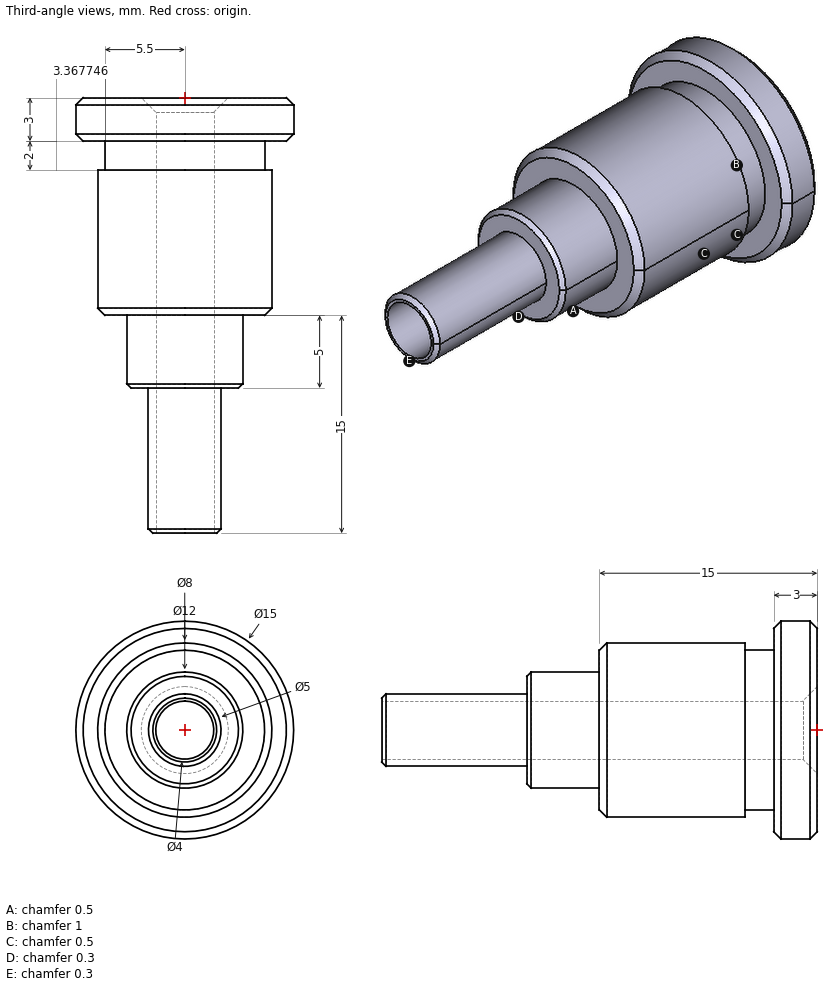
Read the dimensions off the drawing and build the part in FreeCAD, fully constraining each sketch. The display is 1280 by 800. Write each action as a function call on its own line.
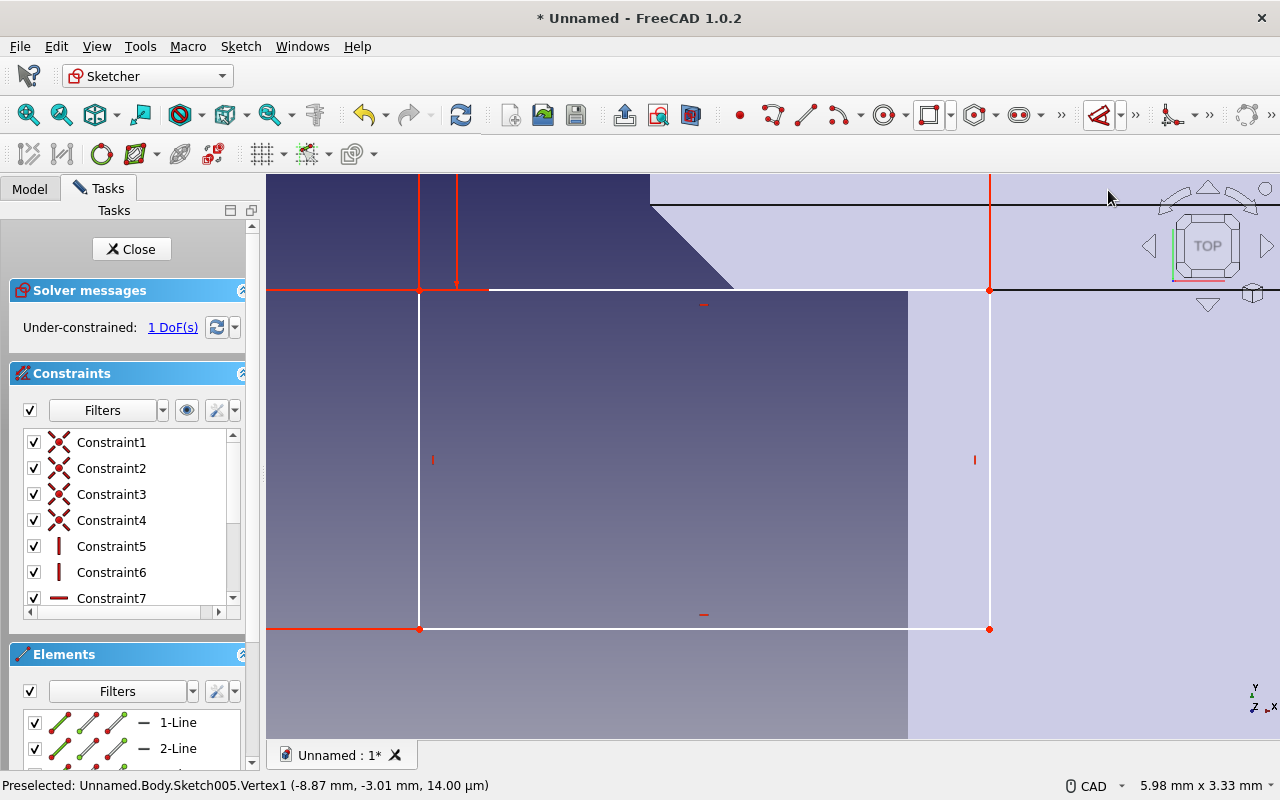
click(990, 629)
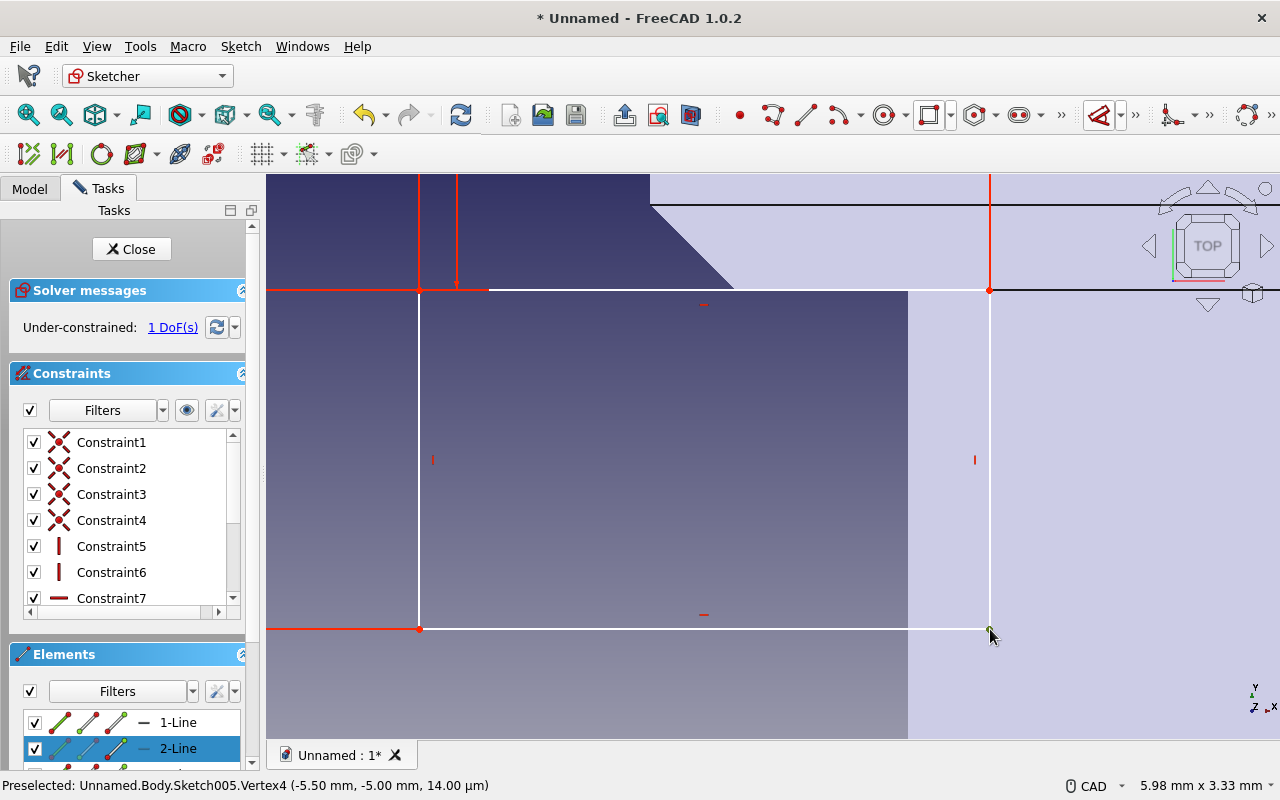
key(l)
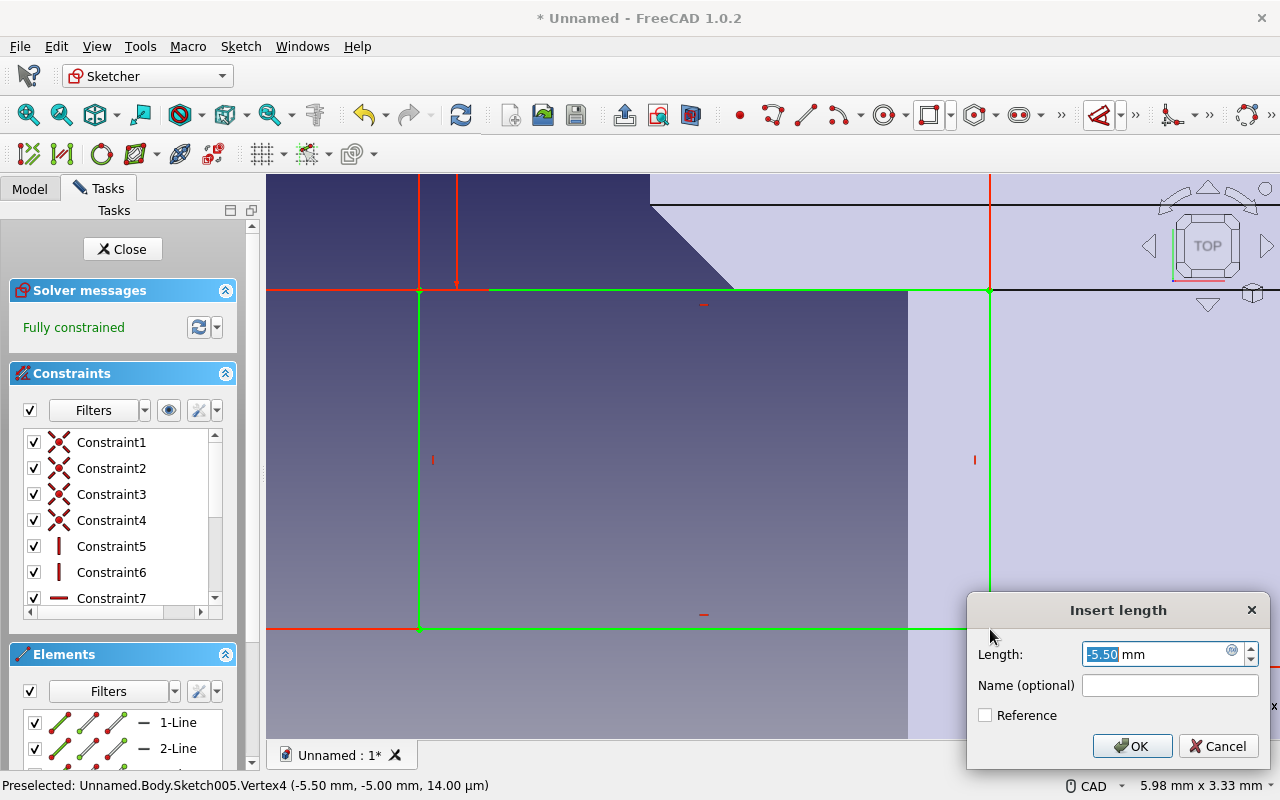
text(-5.5)
key(Return)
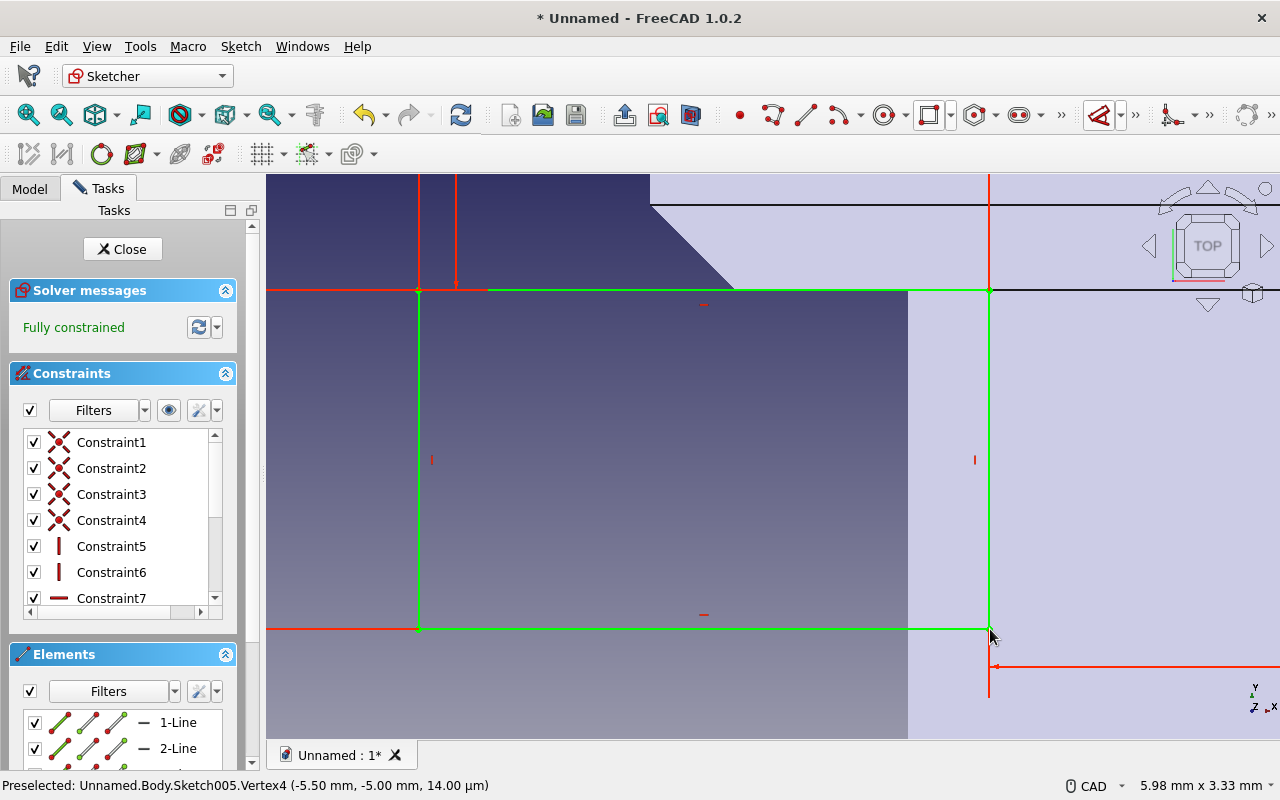
click(123, 249)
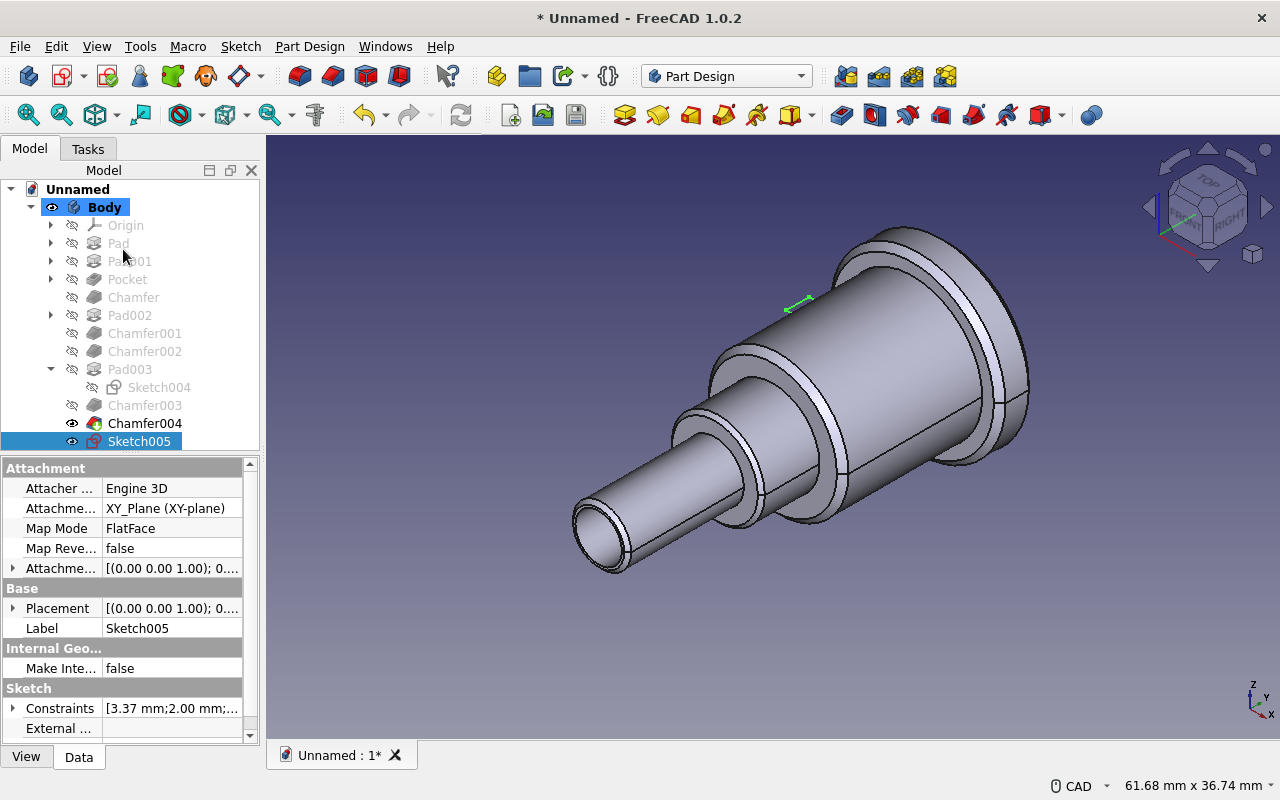
click(908, 116)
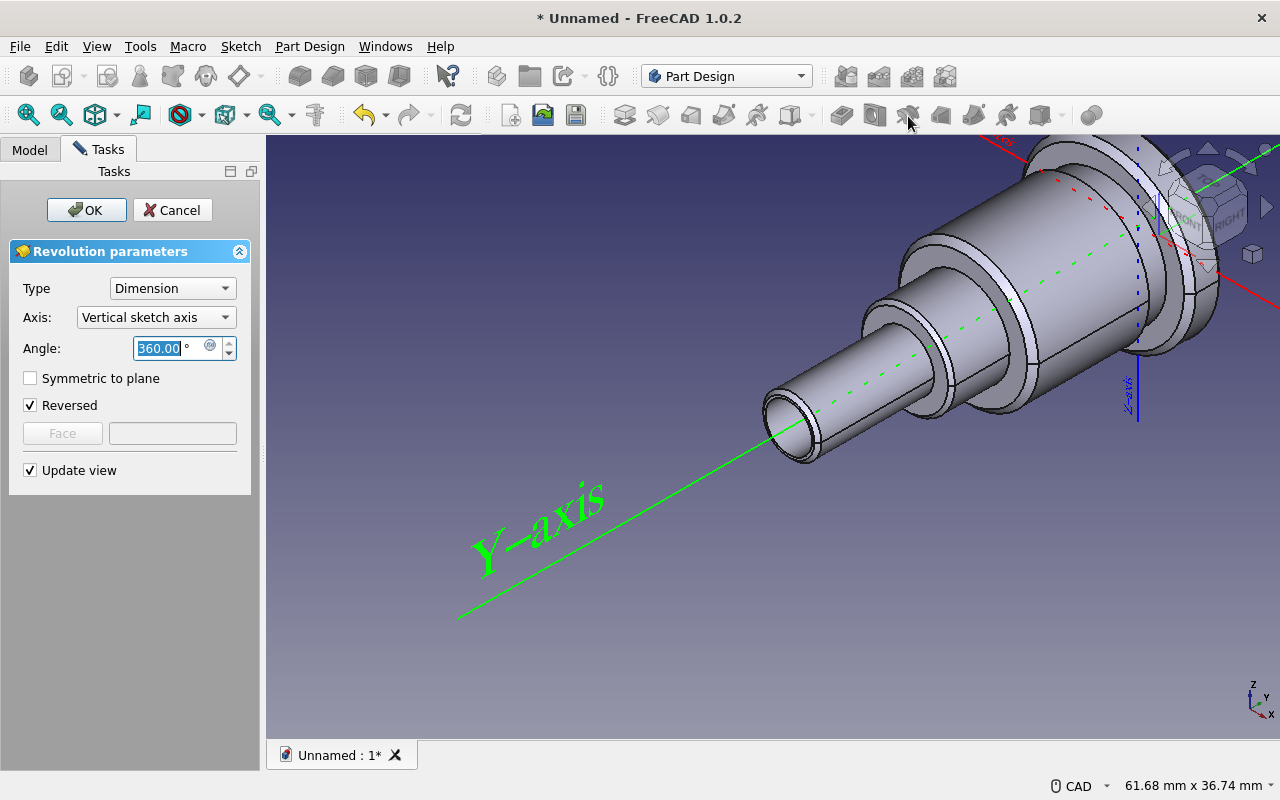
click(87, 210)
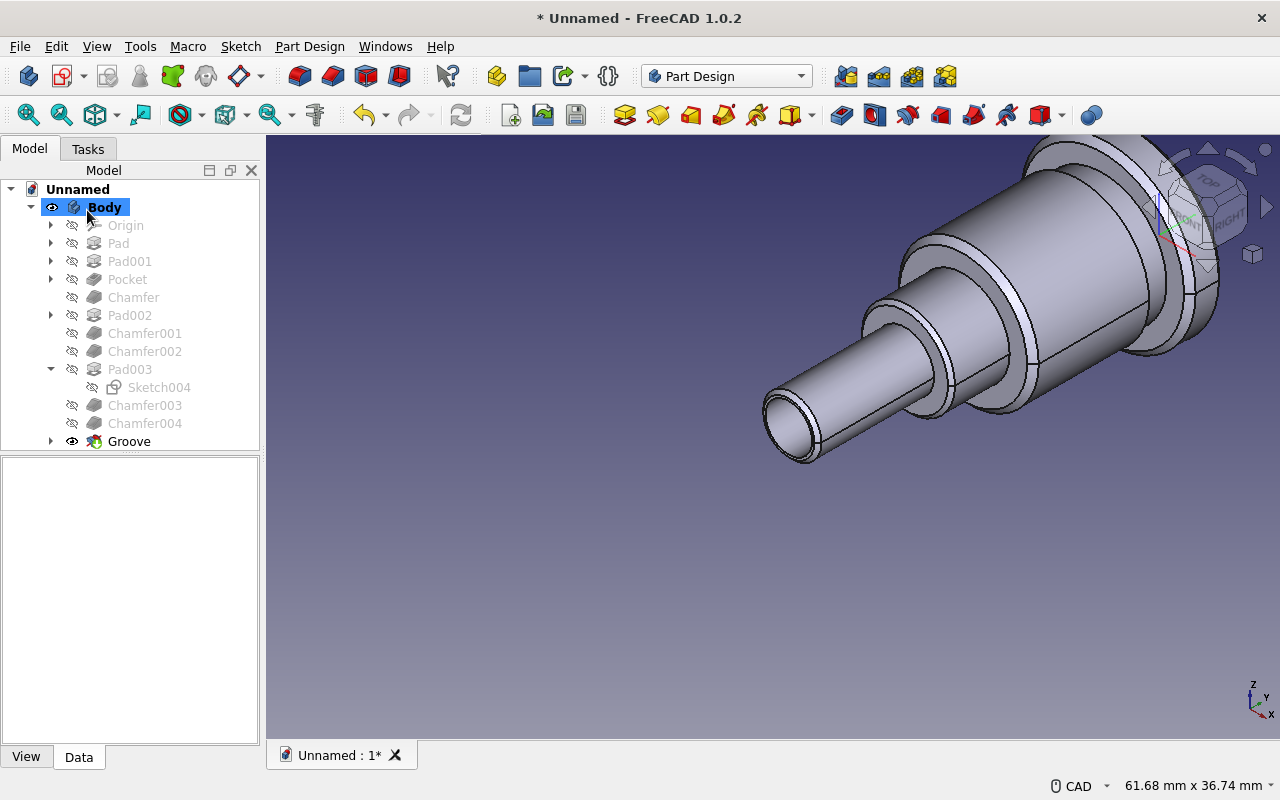
click(29, 116)